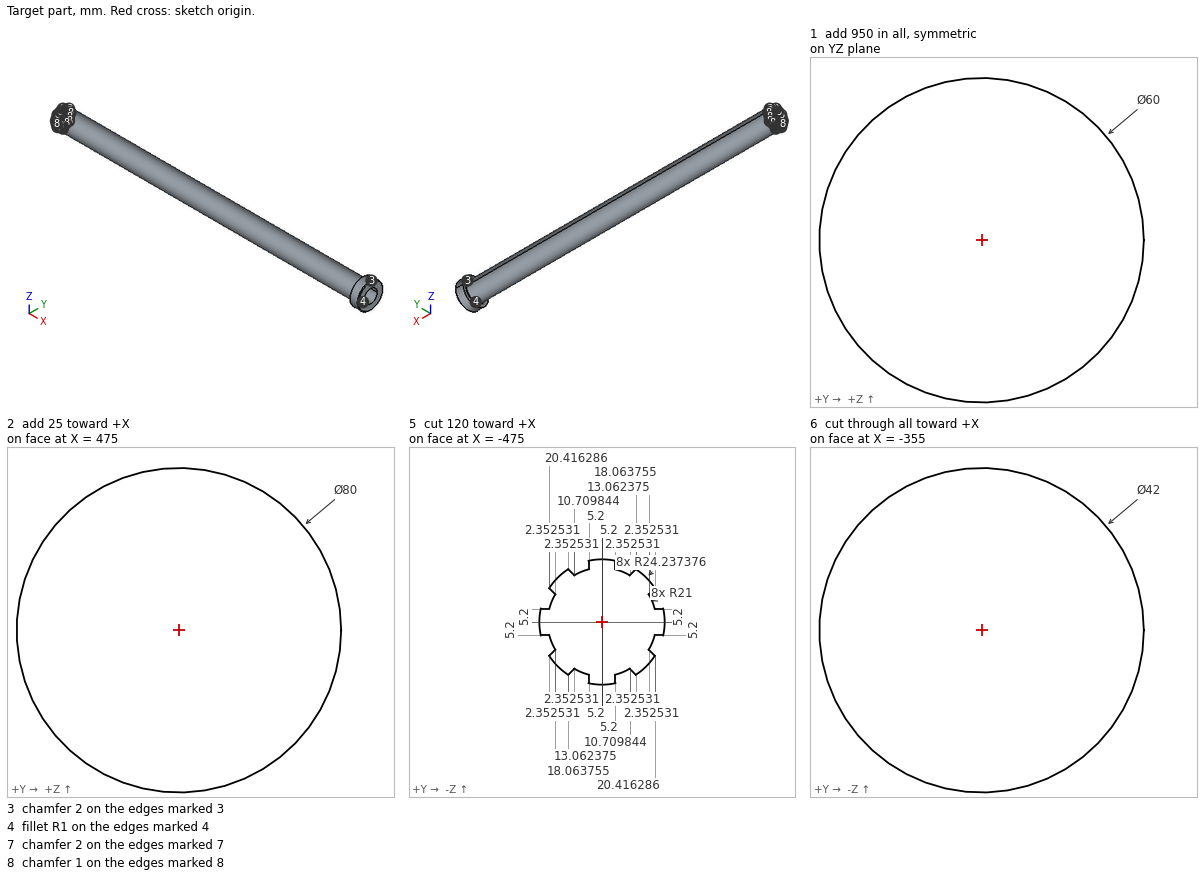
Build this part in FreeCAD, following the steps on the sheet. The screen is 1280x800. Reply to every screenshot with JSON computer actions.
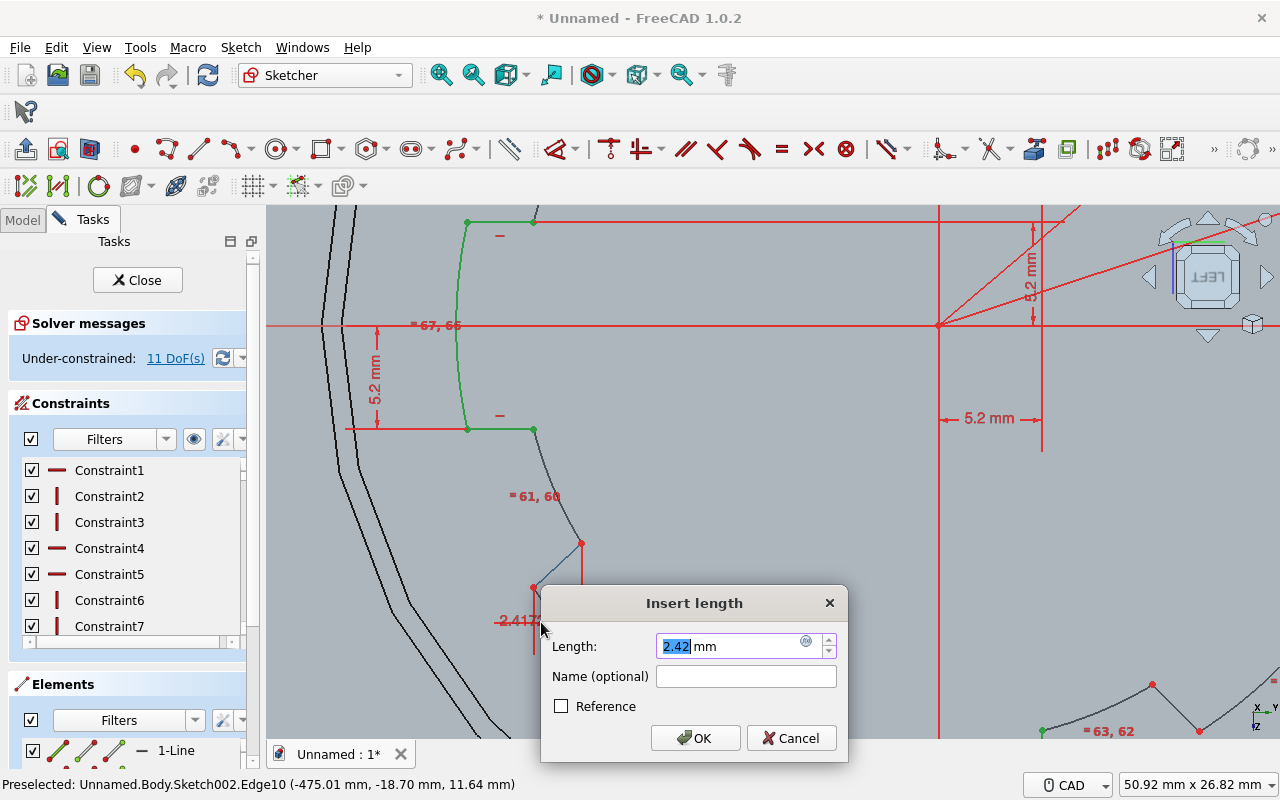
{"action": "type", "text": "2.352531"}
{"action": "key", "text": "Return"}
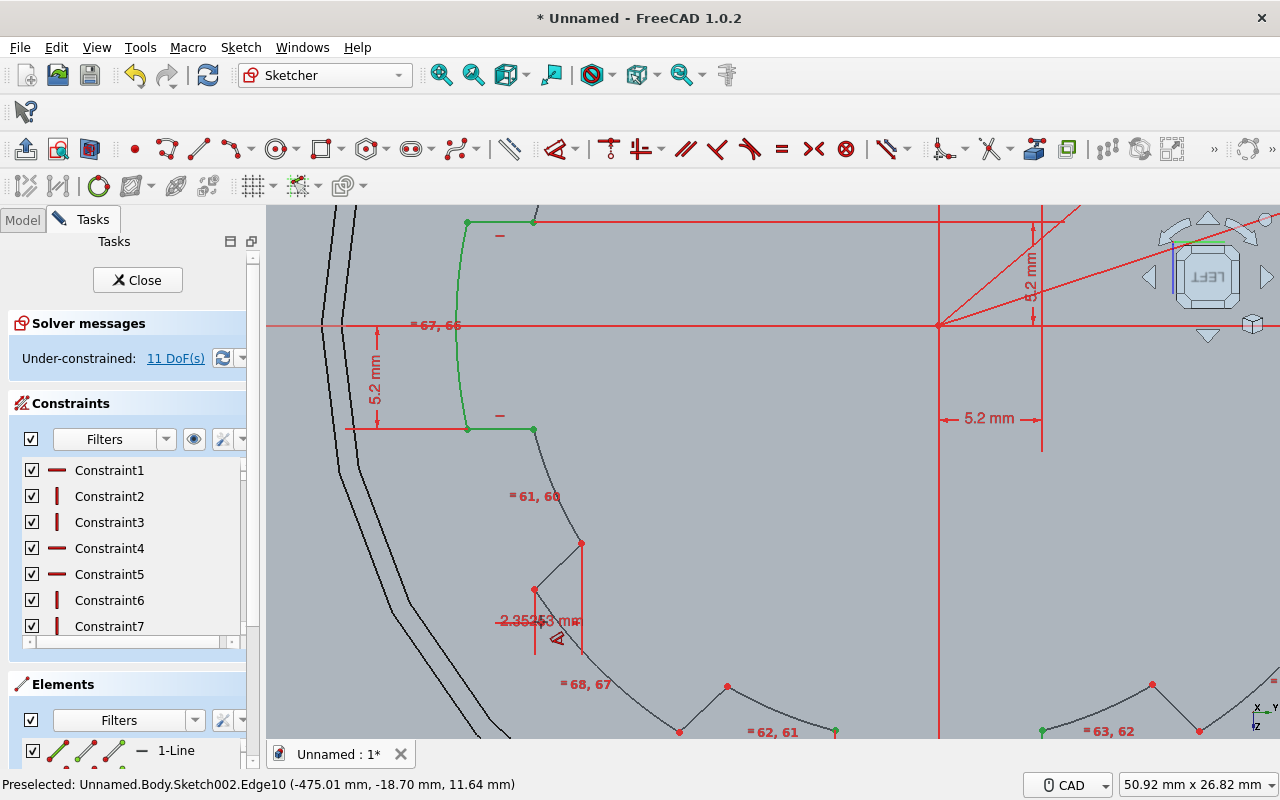
{"action": "left_click", "coordinate": [713, 700]}
{"action": "left_click", "coordinate": [704, 653]}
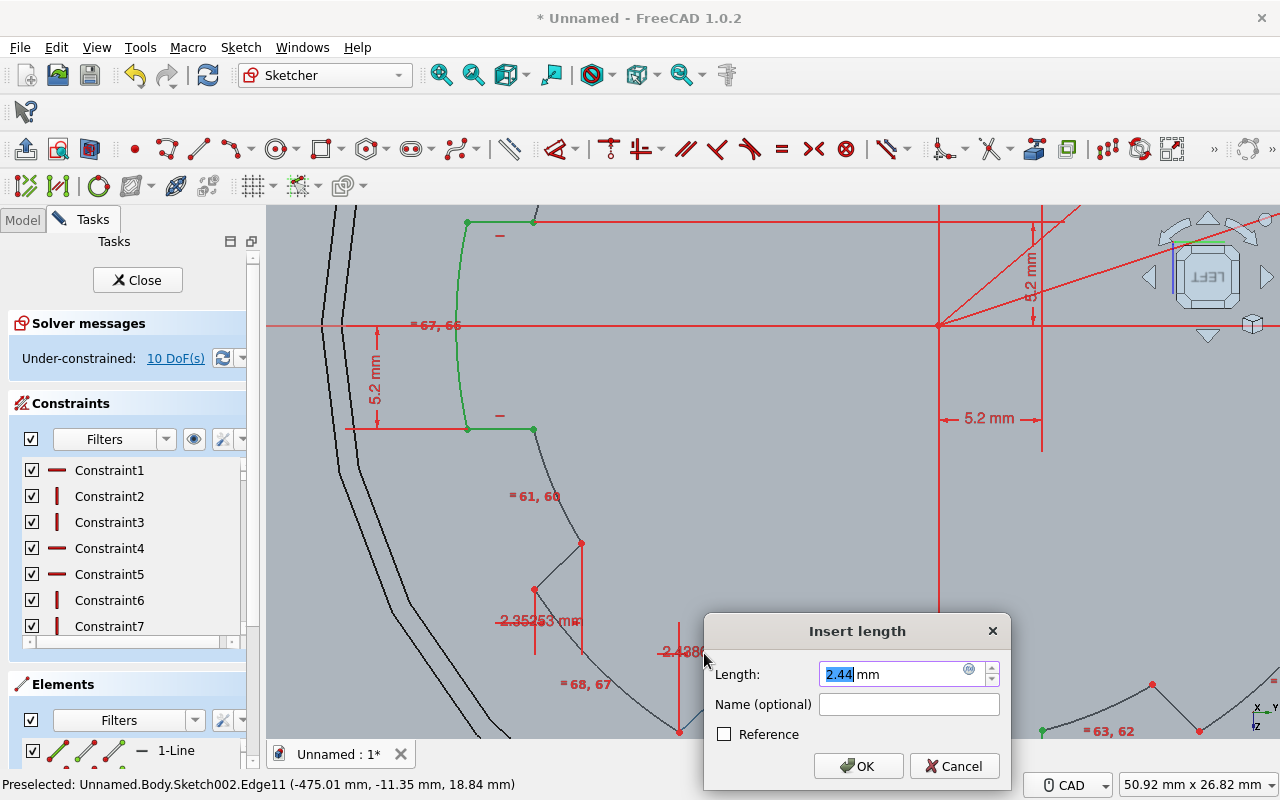
{"action": "type", "text": "2.352531"}
{"action": "key", "text": "Return"}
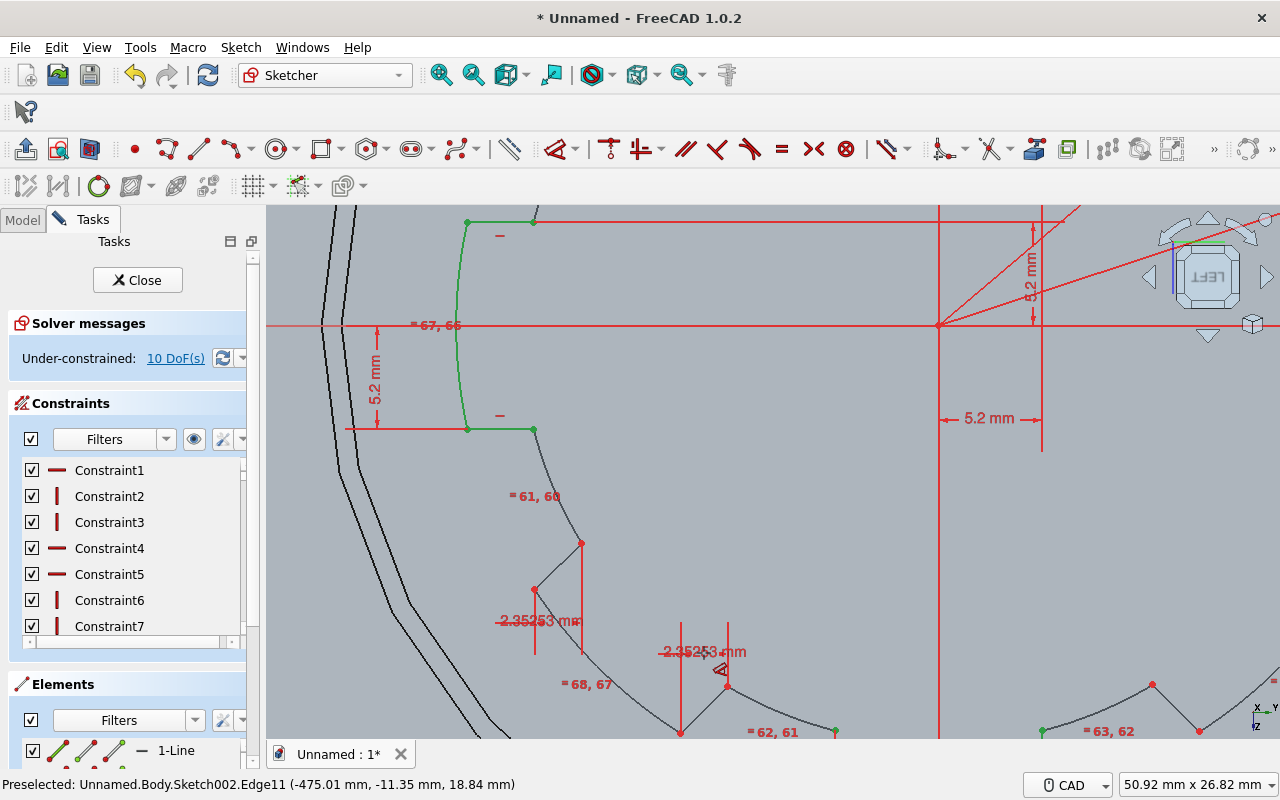
{"action": "scroll", "coordinate": [568, 557], "scroll_direction": "down", "scroll_amount": 5}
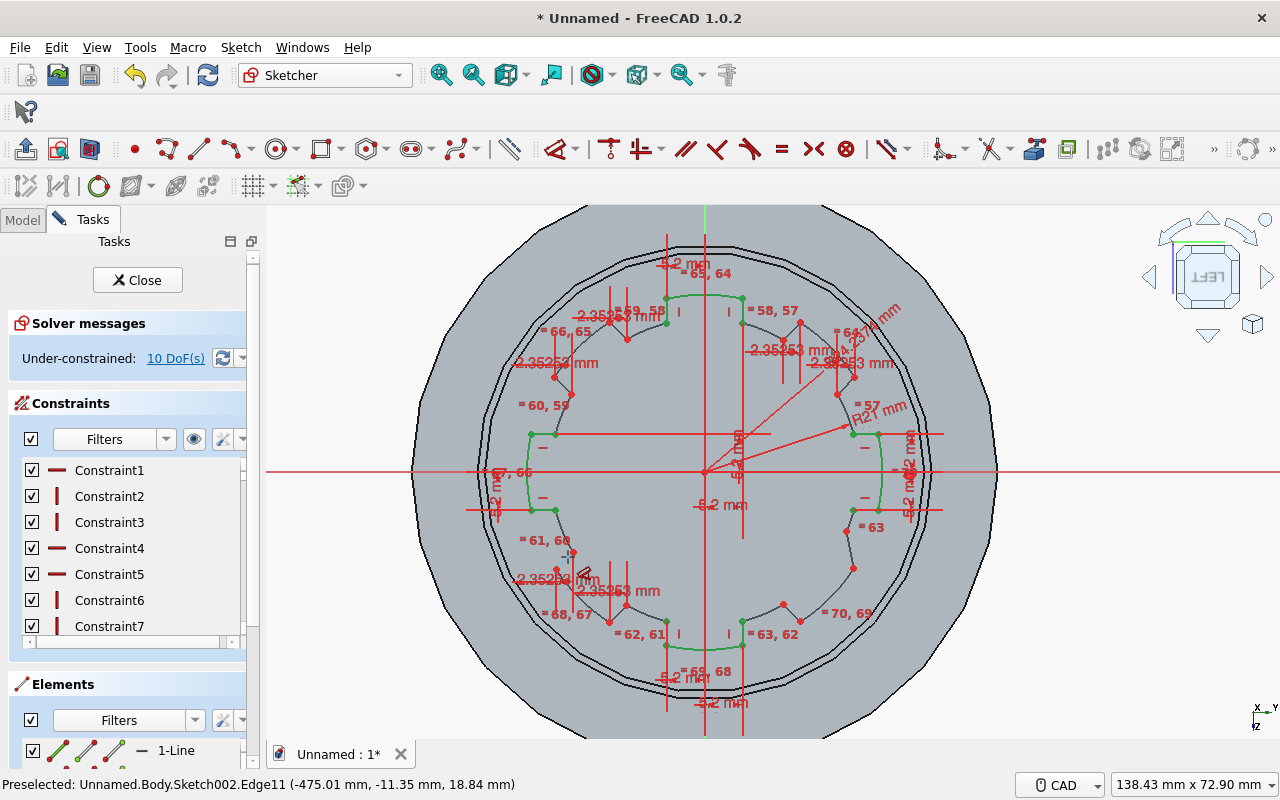
{"action": "scroll", "coordinate": [788, 610], "scroll_direction": "up", "scroll_amount": 5}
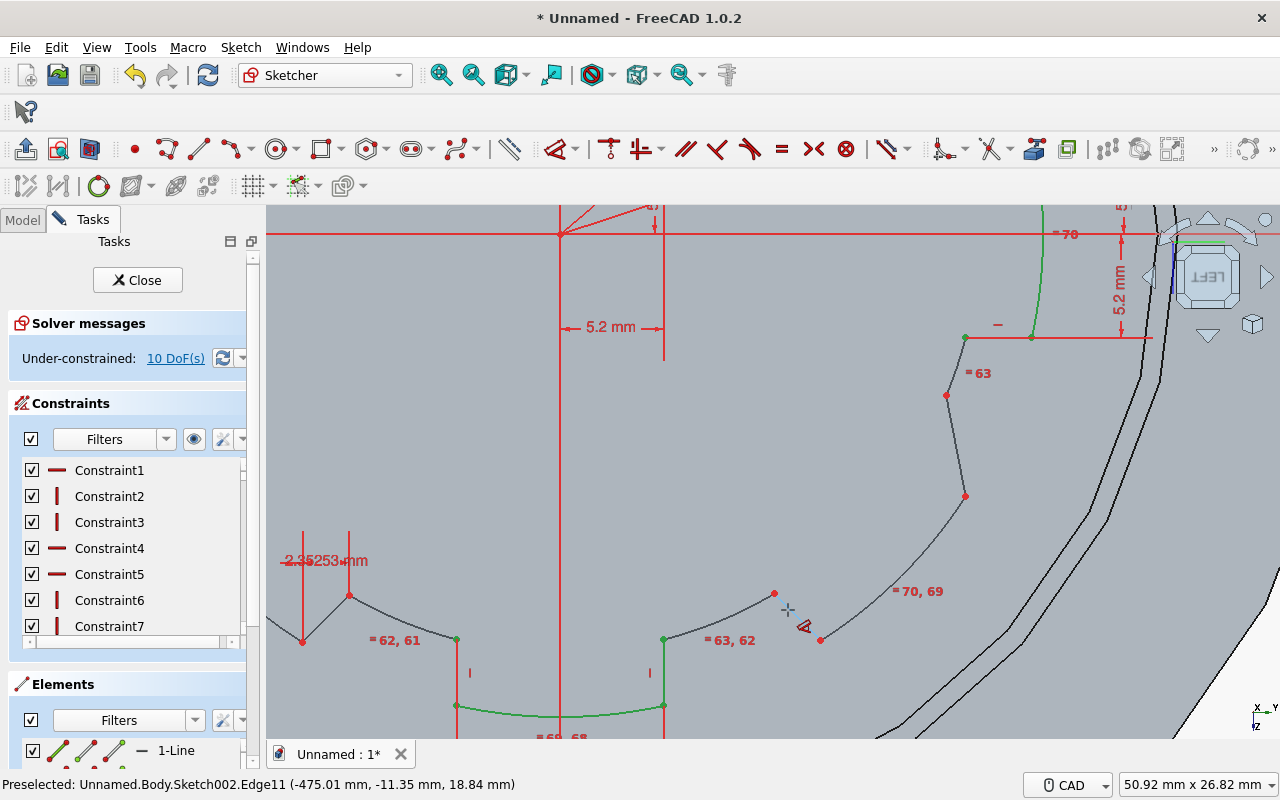
{"action": "left_click", "coordinate": [788, 608]}
{"action": "left_click", "coordinate": [798, 675]}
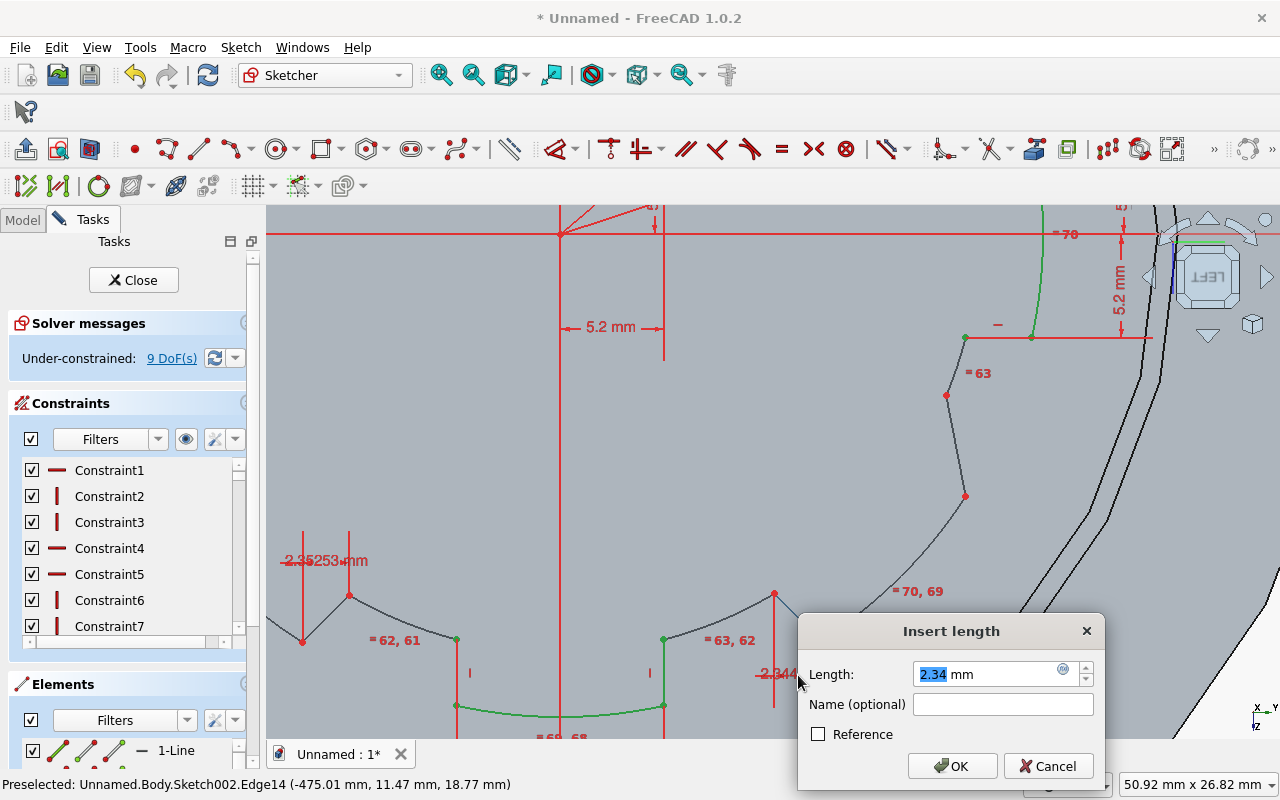
{"action": "type", "text": "2.352531"}
{"action": "key", "text": "Return"}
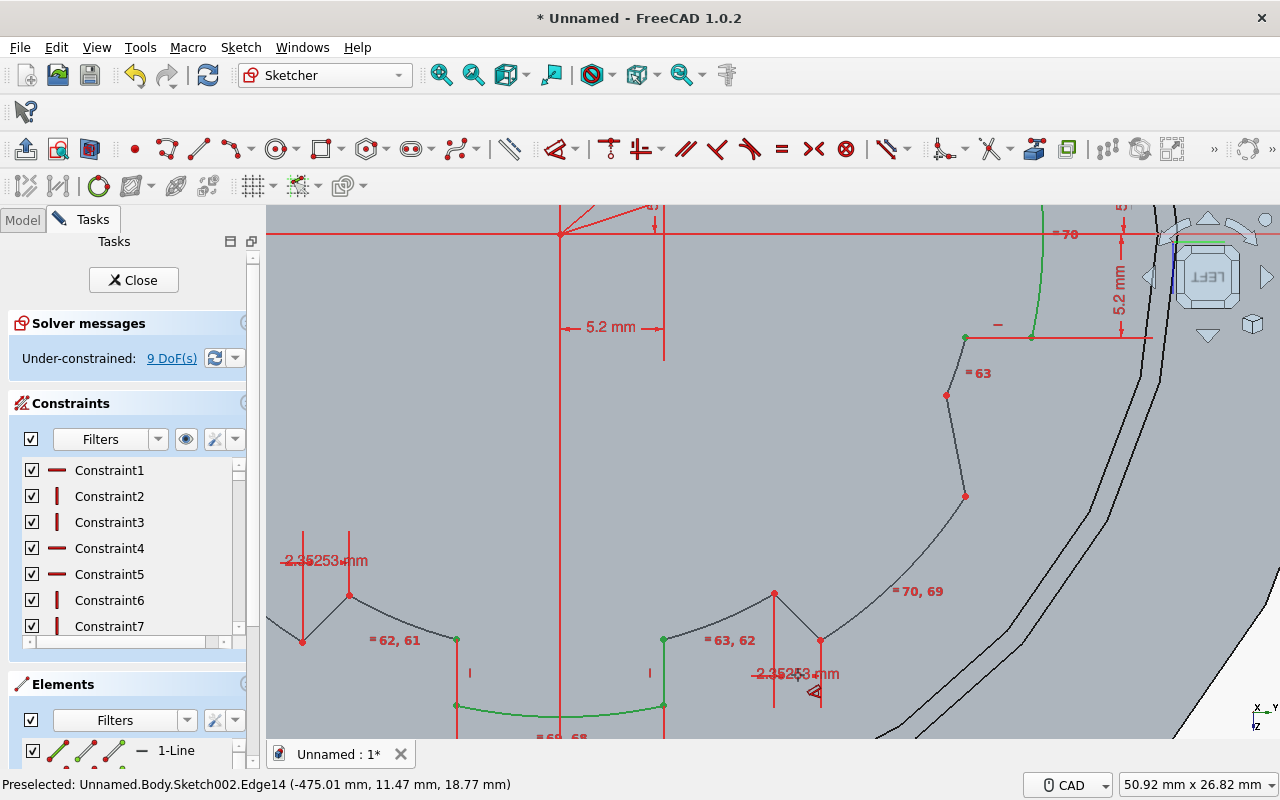
{"action": "left_click", "coordinate": [960, 466]}
{"action": "left_click", "coordinate": [960, 530]}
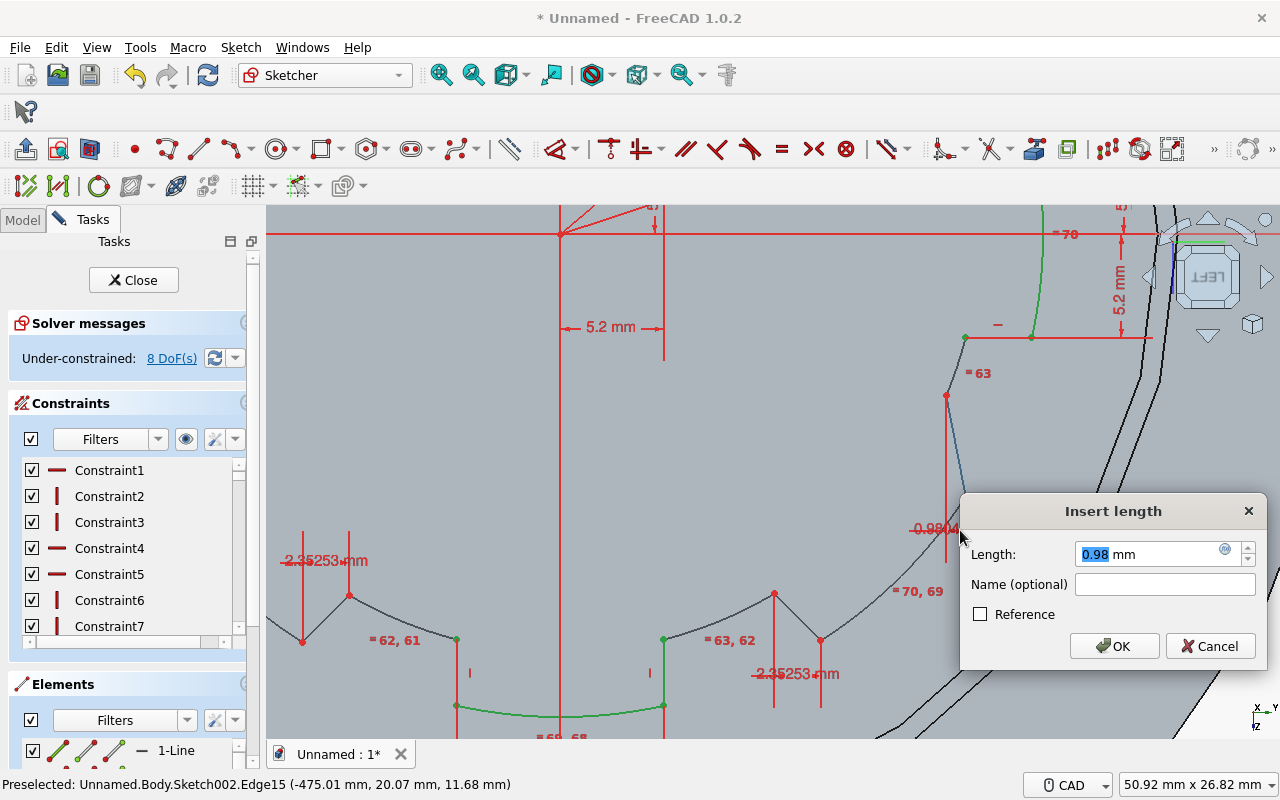
{"action": "type", "text": "2.352531"}
{"action": "key", "text": "Return"}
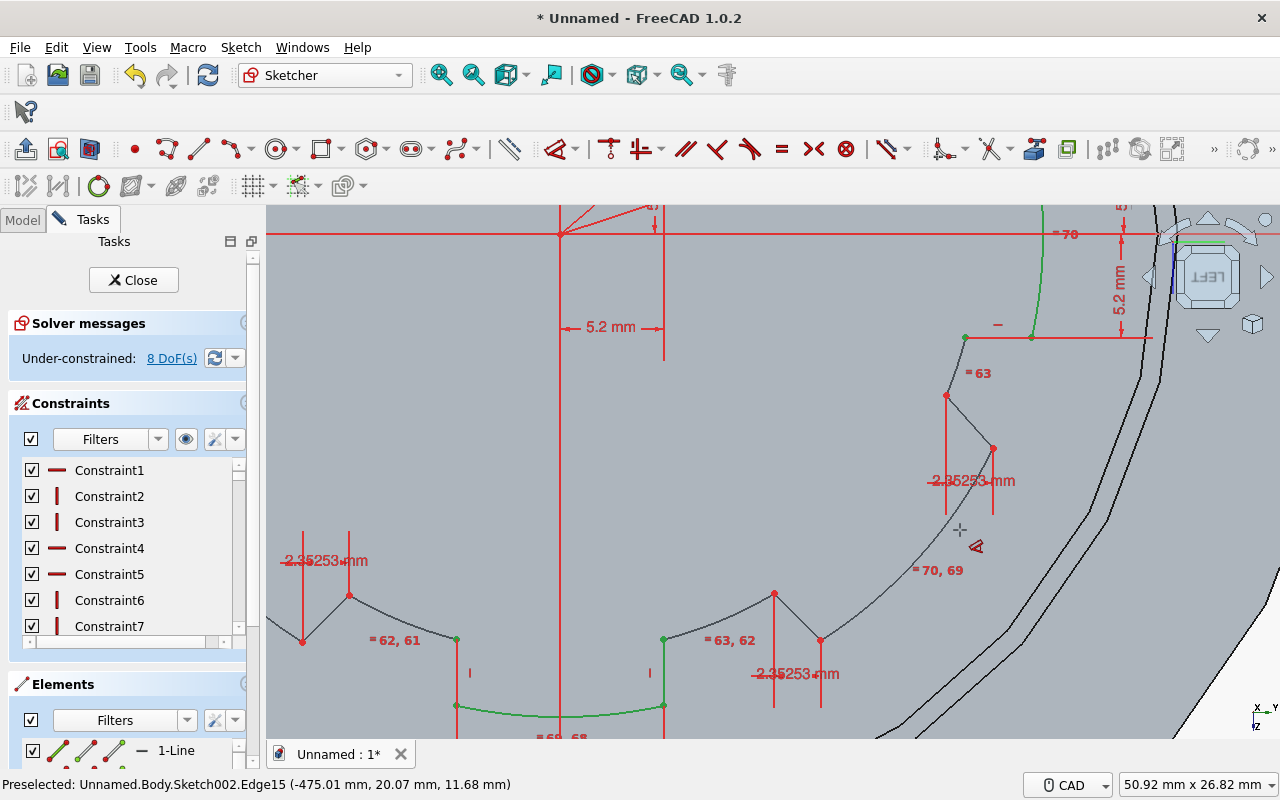
{"action": "scroll", "coordinate": [788, 610], "scroll_direction": "down", "scroll_amount": 5}